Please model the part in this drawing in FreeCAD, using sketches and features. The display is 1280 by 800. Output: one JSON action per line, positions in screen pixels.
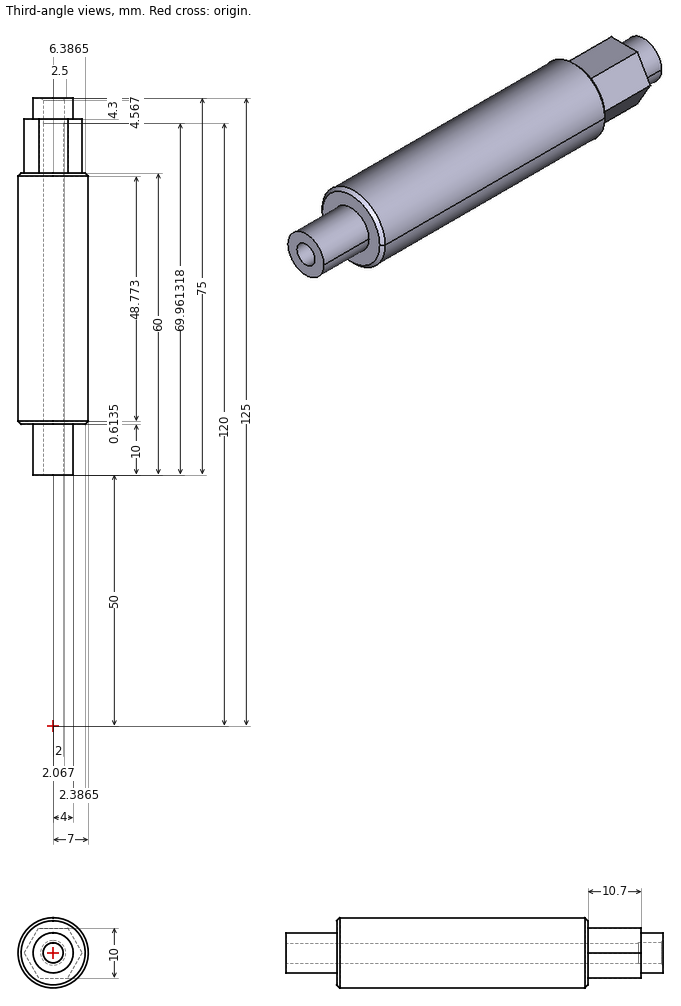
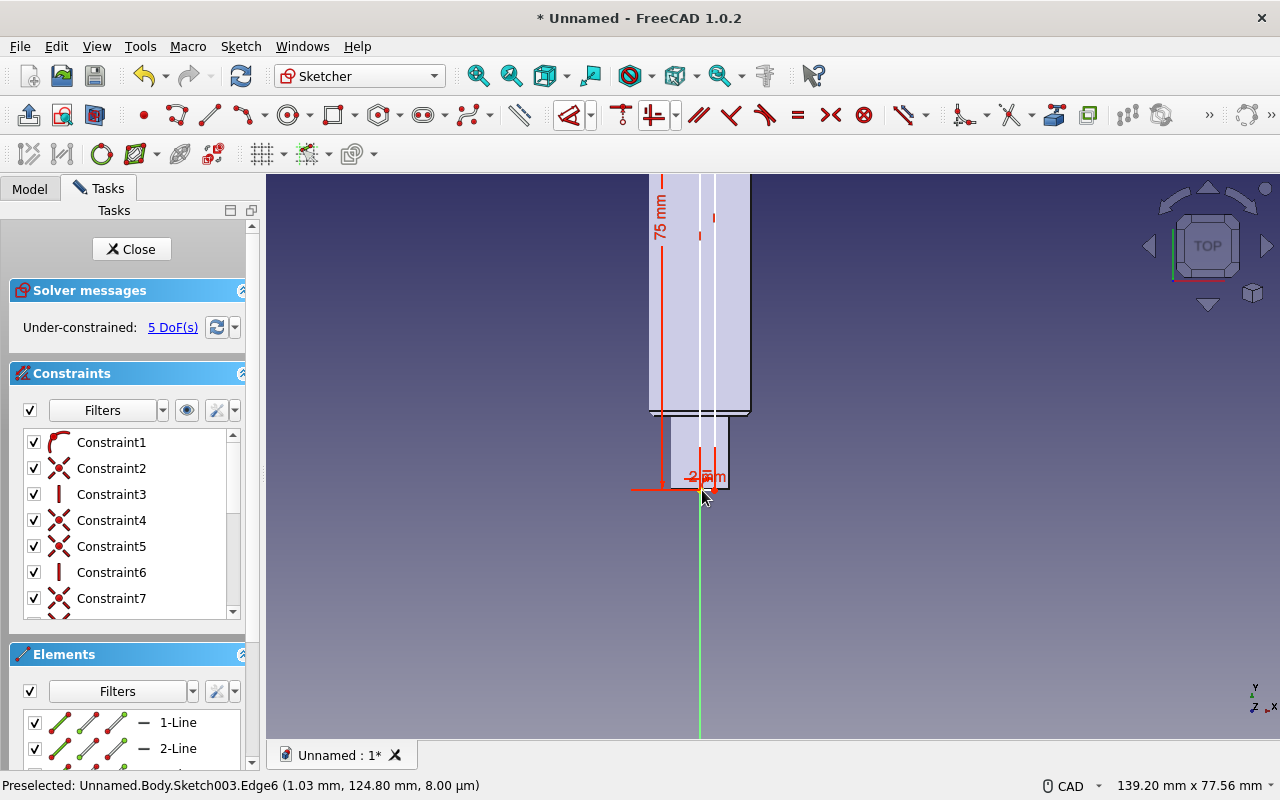
{"action": "left_click", "coordinate": [700, 490]}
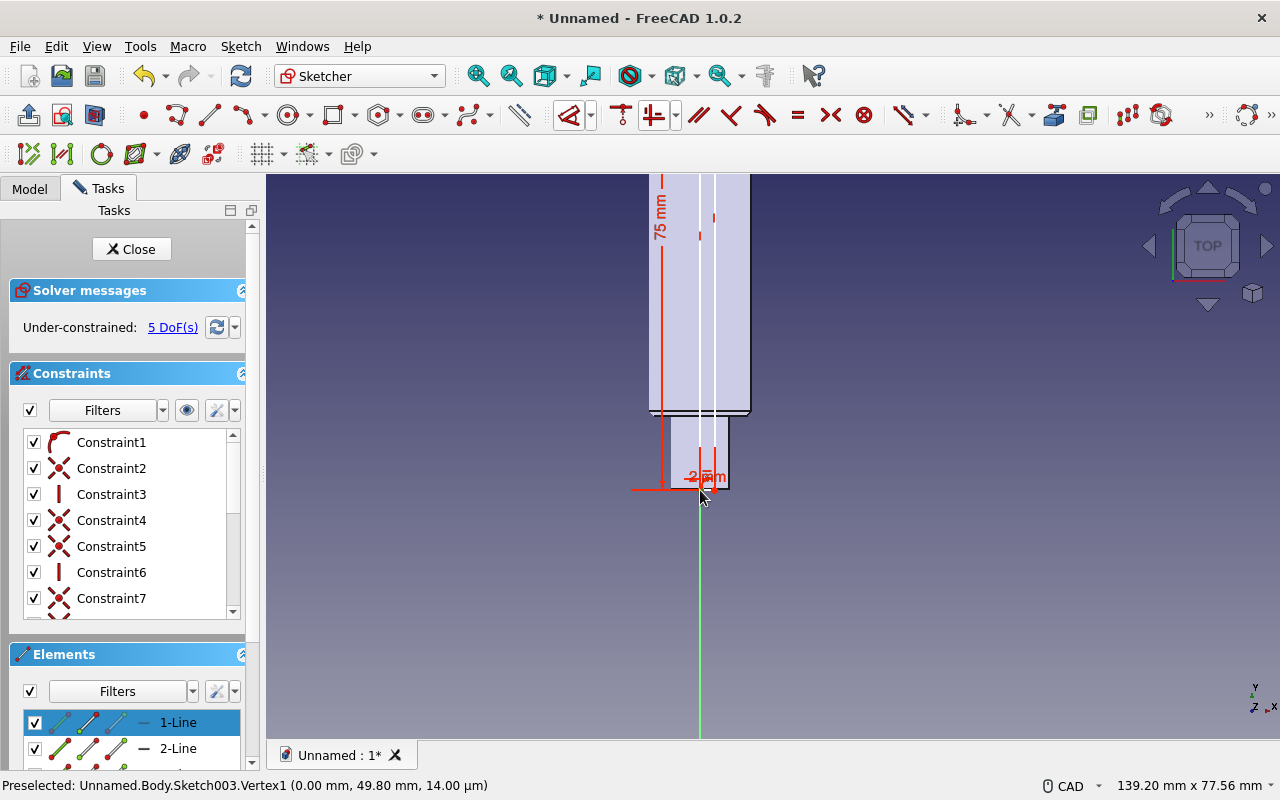
{"action": "left_click", "coordinate": [590, 116]}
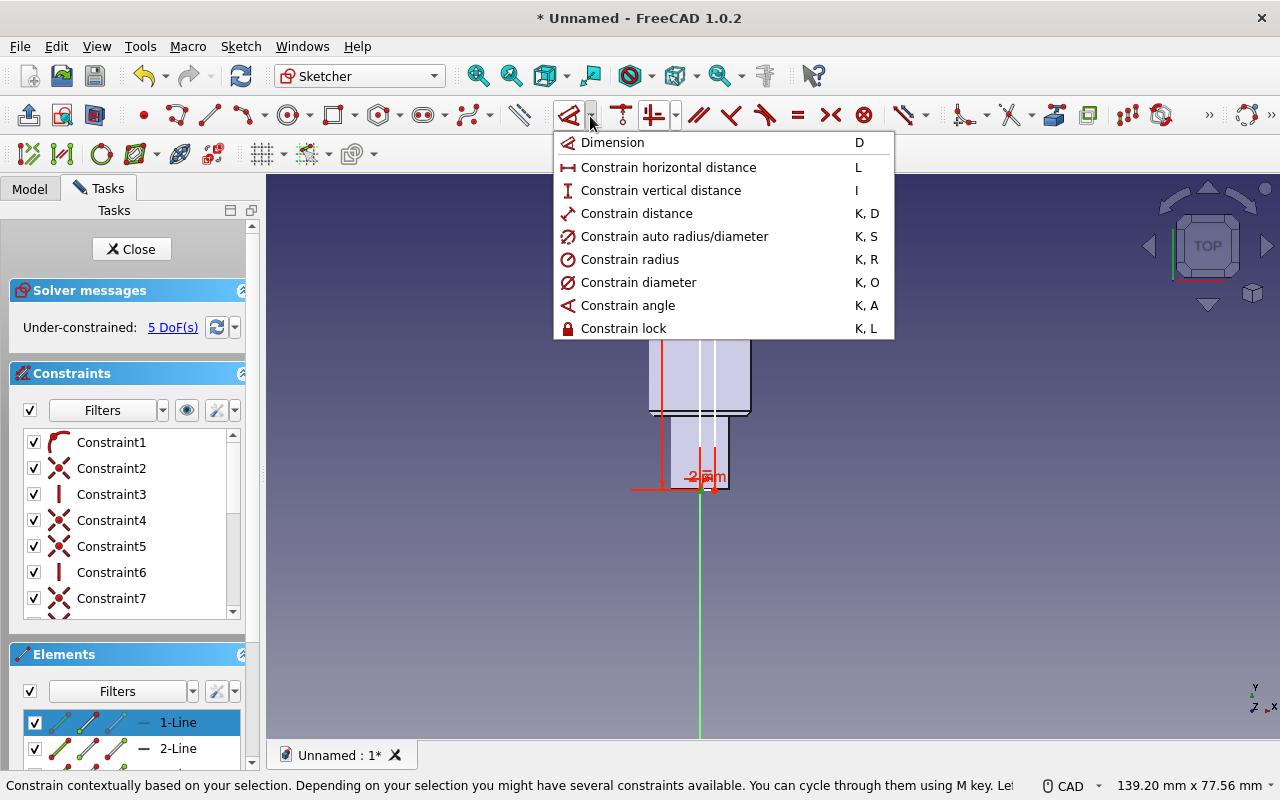
{"action": "left_click", "coordinate": [724, 190]}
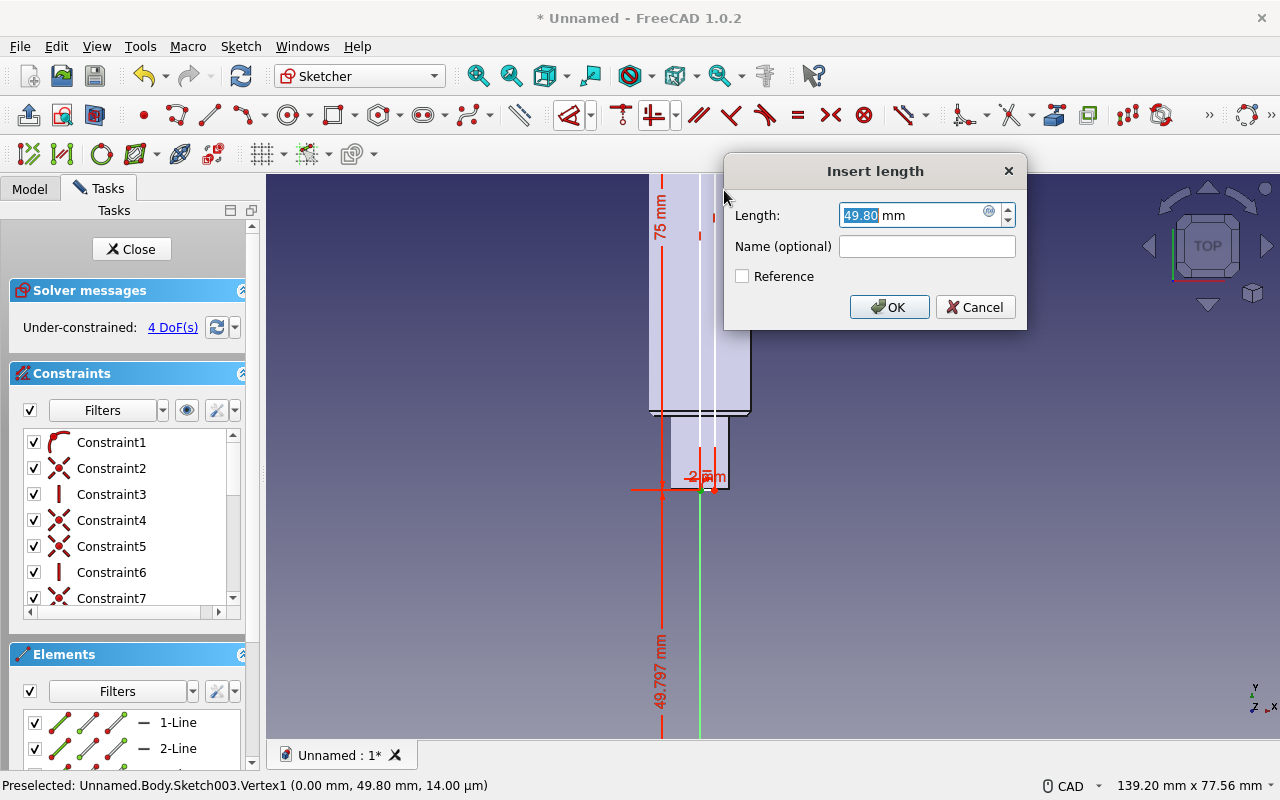
{"action": "type", "text": "50"}
{"action": "key", "text": "Return"}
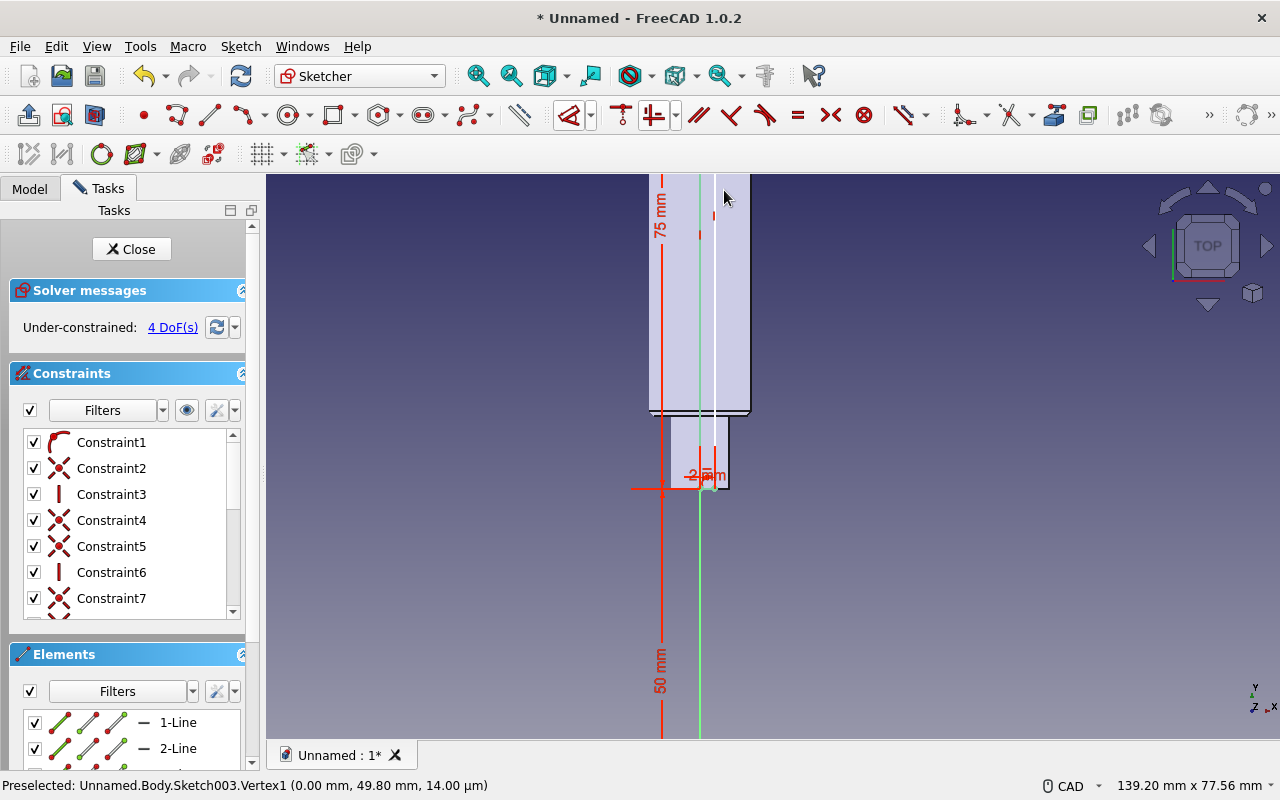
{"action": "scroll", "coordinate": [702, 491], "scroll_direction": "down", "scroll_amount": 5}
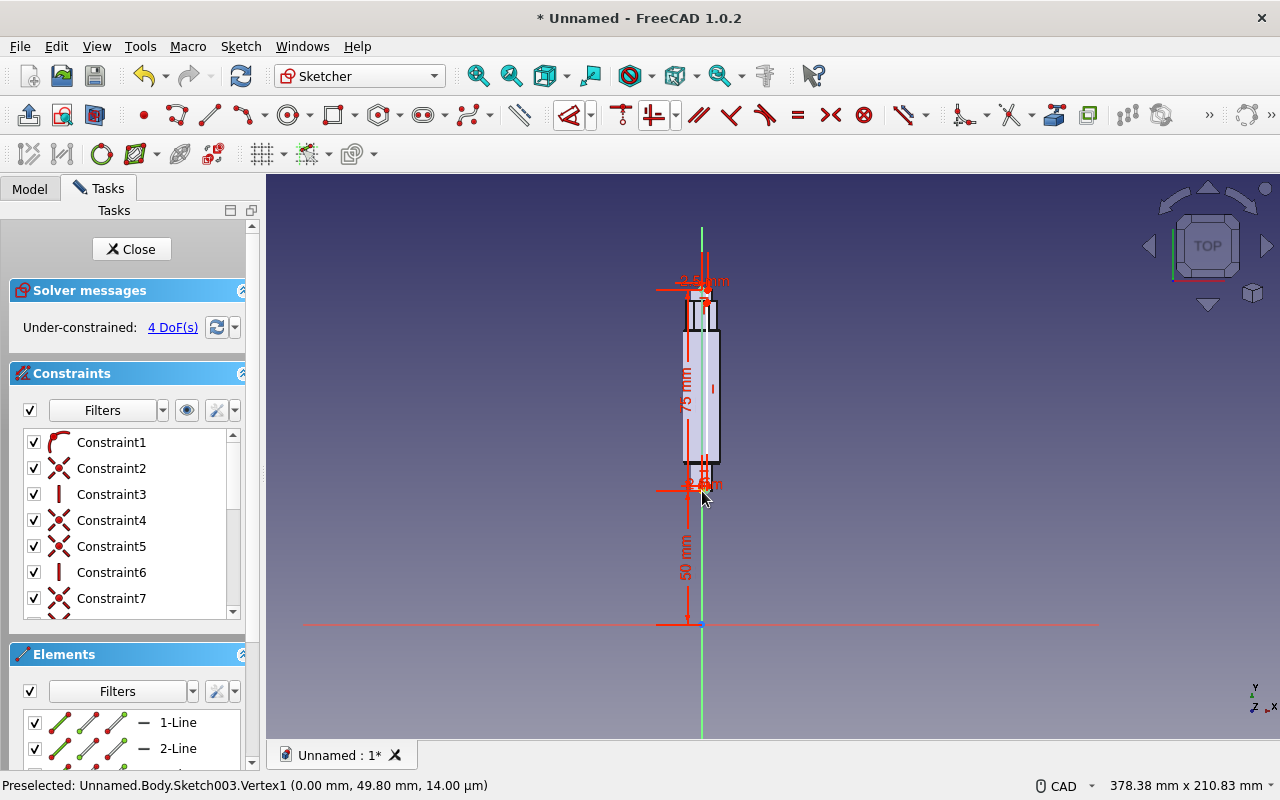
{"action": "scroll", "coordinate": [707, 303], "scroll_direction": "up", "scroll_amount": 14}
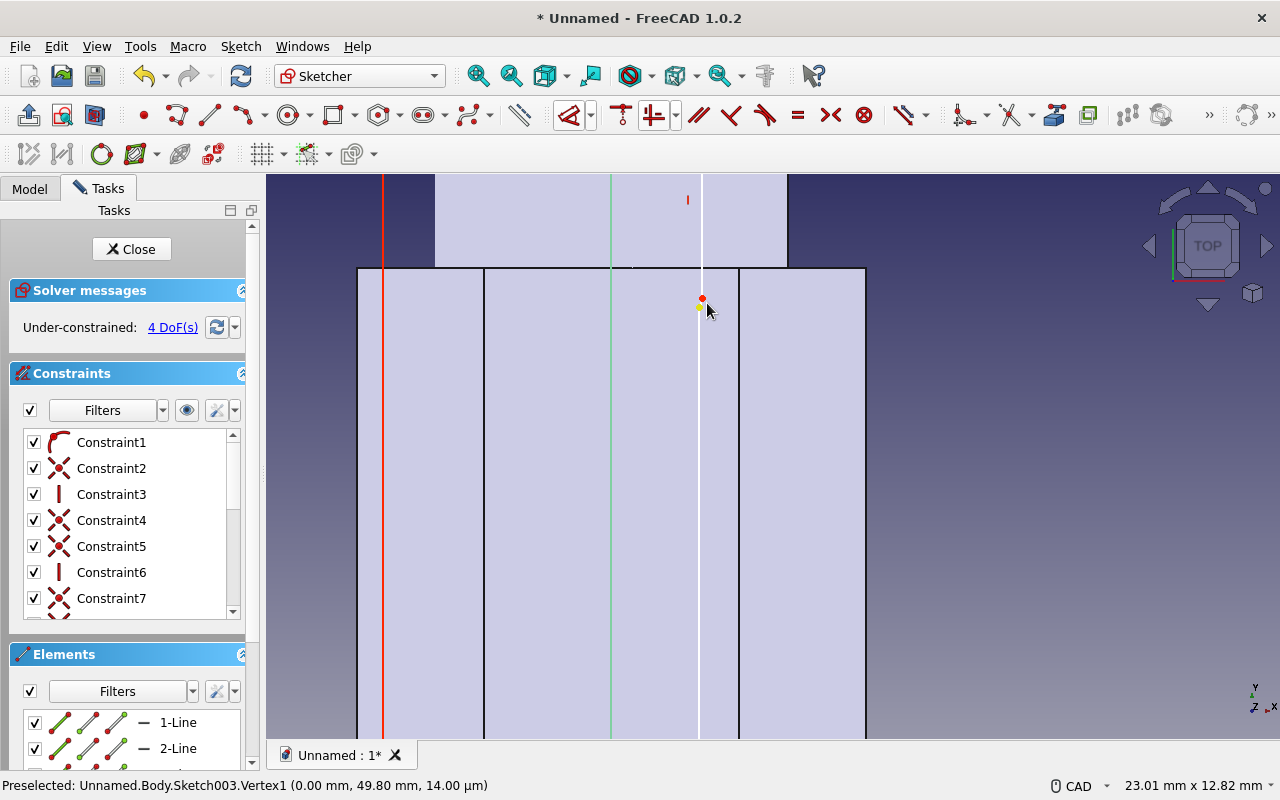
{"action": "left_click", "coordinate": [702, 299]}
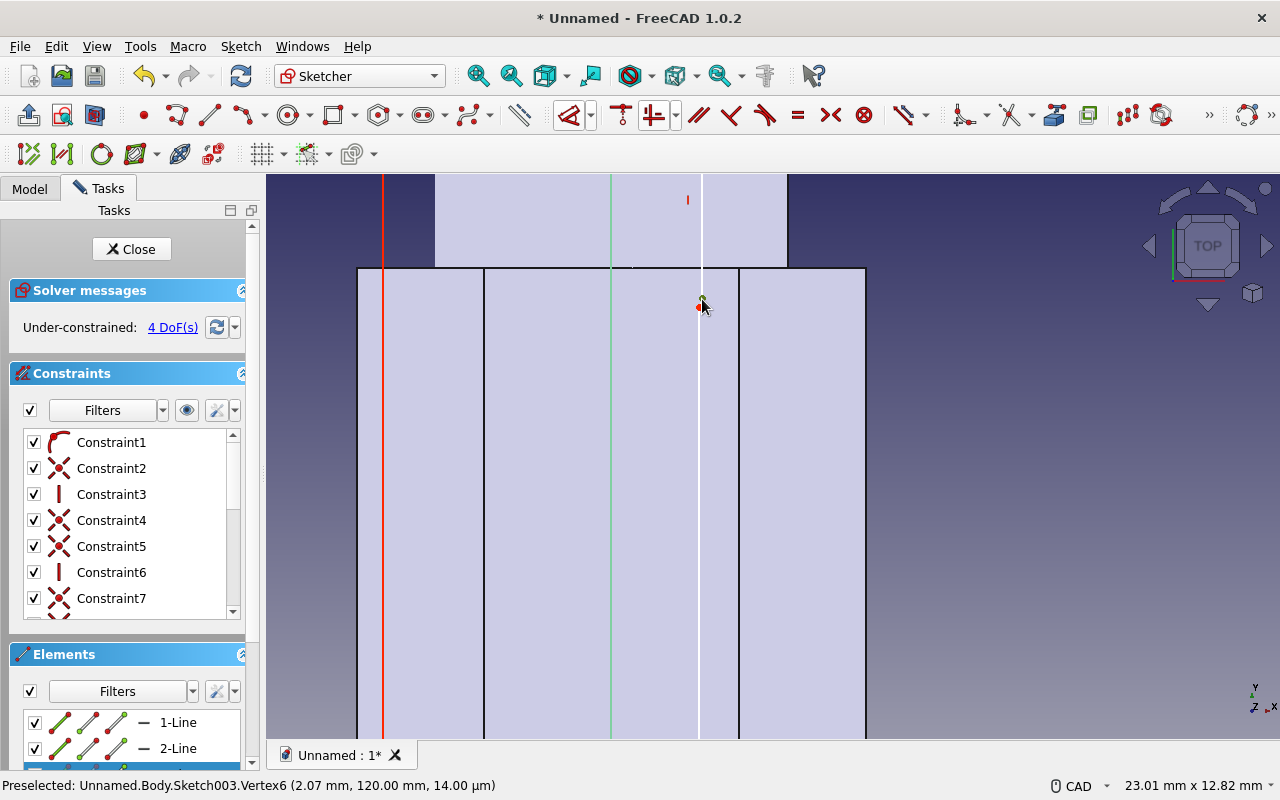
{"action": "left_click", "coordinate": [590, 116]}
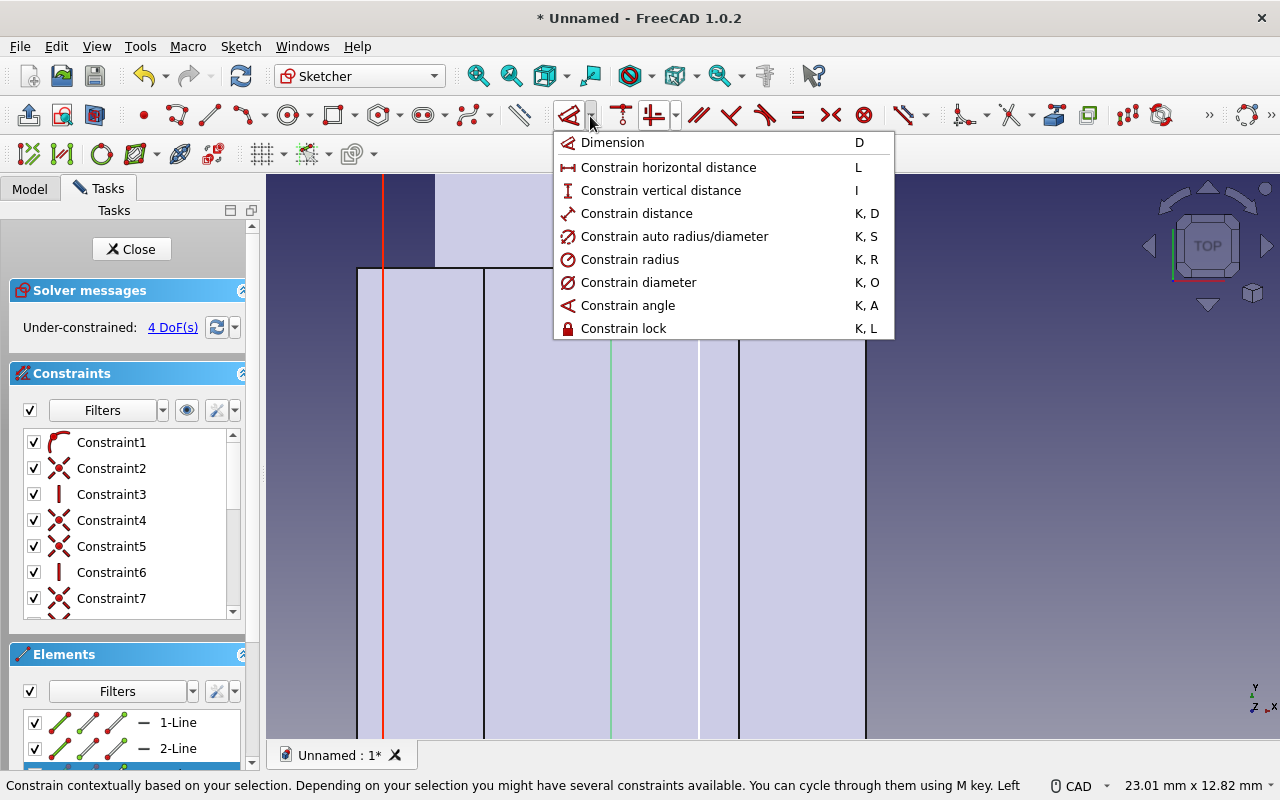
{"action": "left_click", "coordinate": [724, 190]}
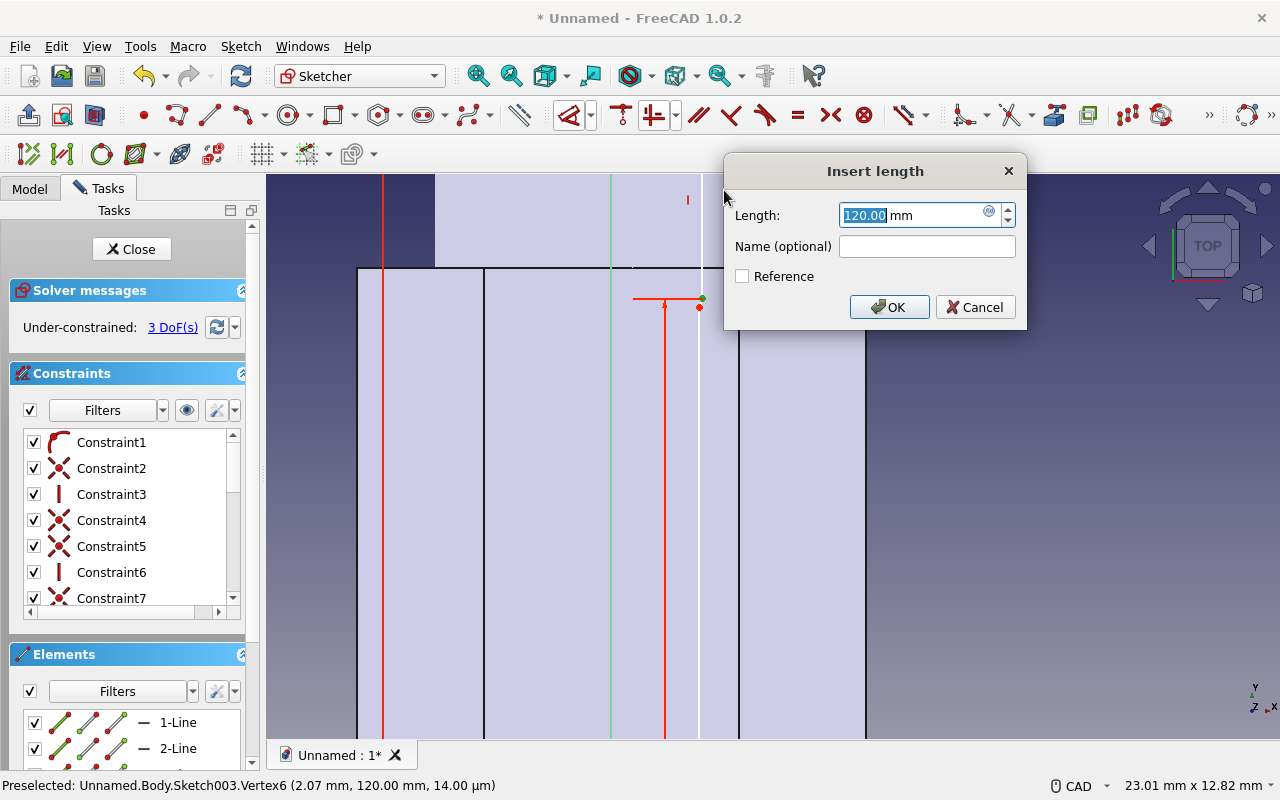
{"action": "type", "text": "120"}
{"action": "key", "text": "Return"}